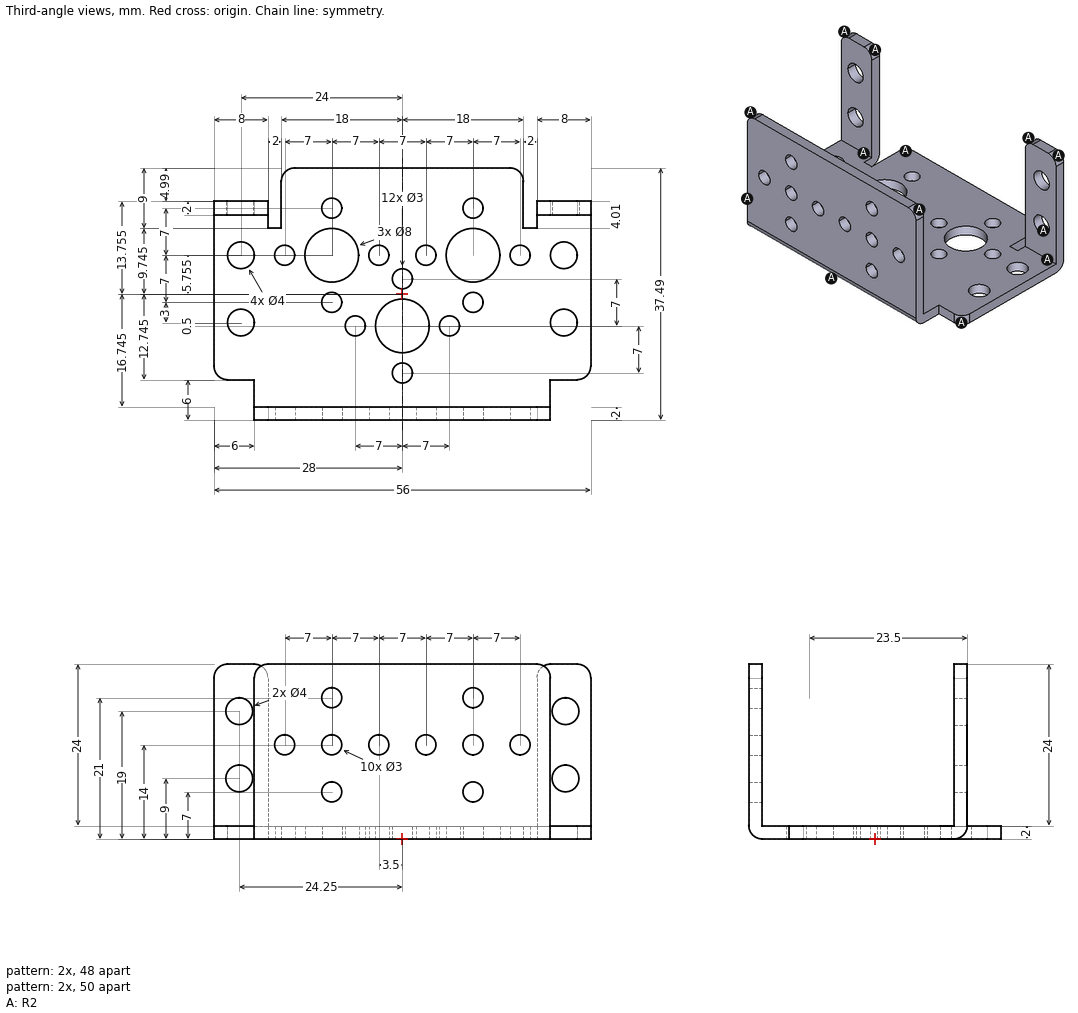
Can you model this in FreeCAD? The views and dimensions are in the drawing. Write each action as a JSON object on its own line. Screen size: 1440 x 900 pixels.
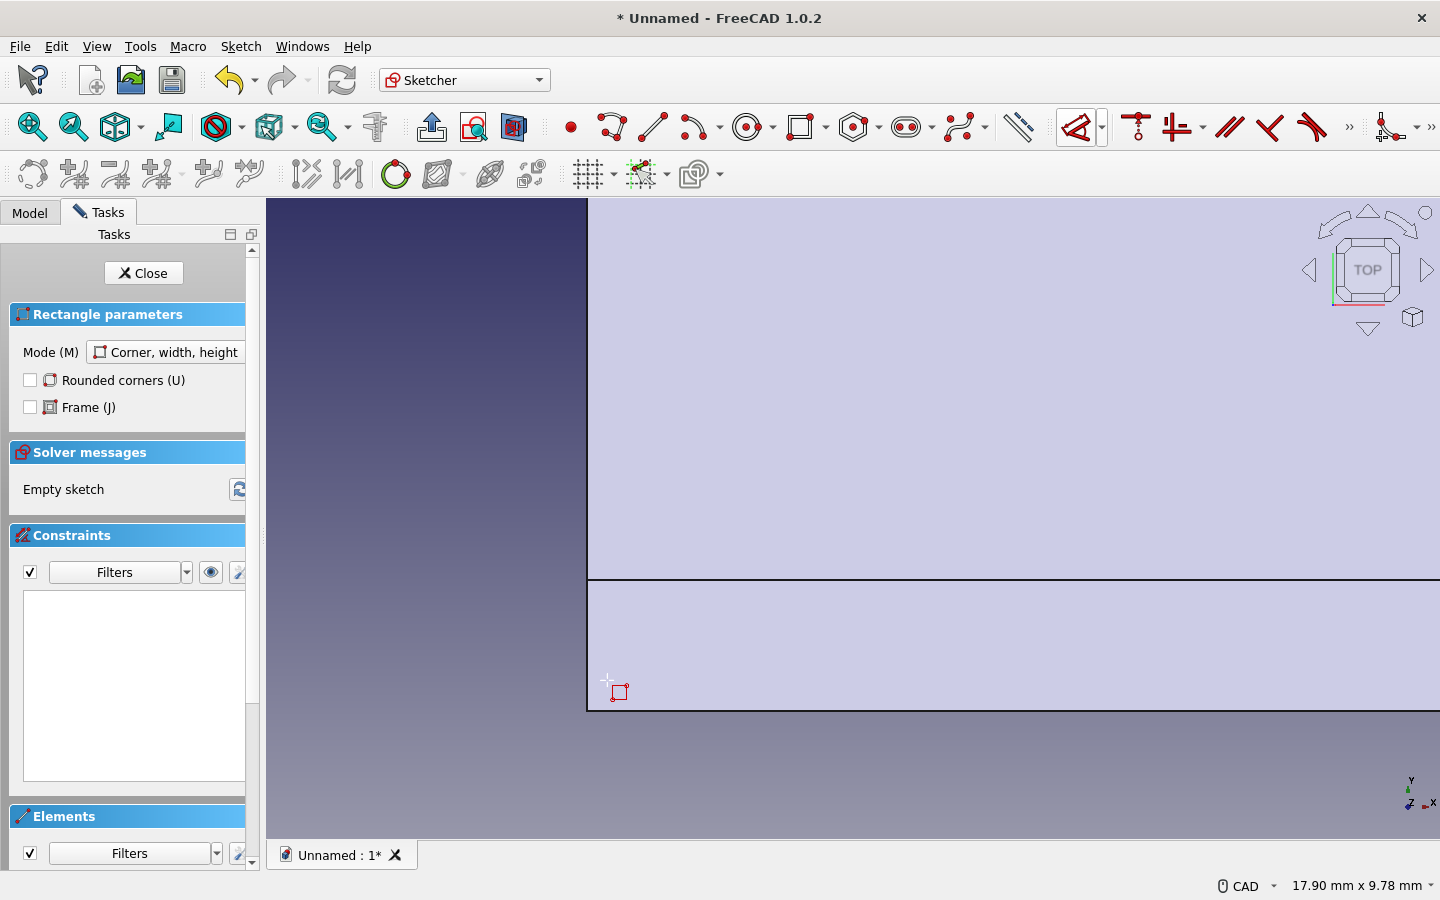
{"action": "left_click", "coordinate": [587, 318]}
{"action": "mouse_move", "coordinate": [980, 711]}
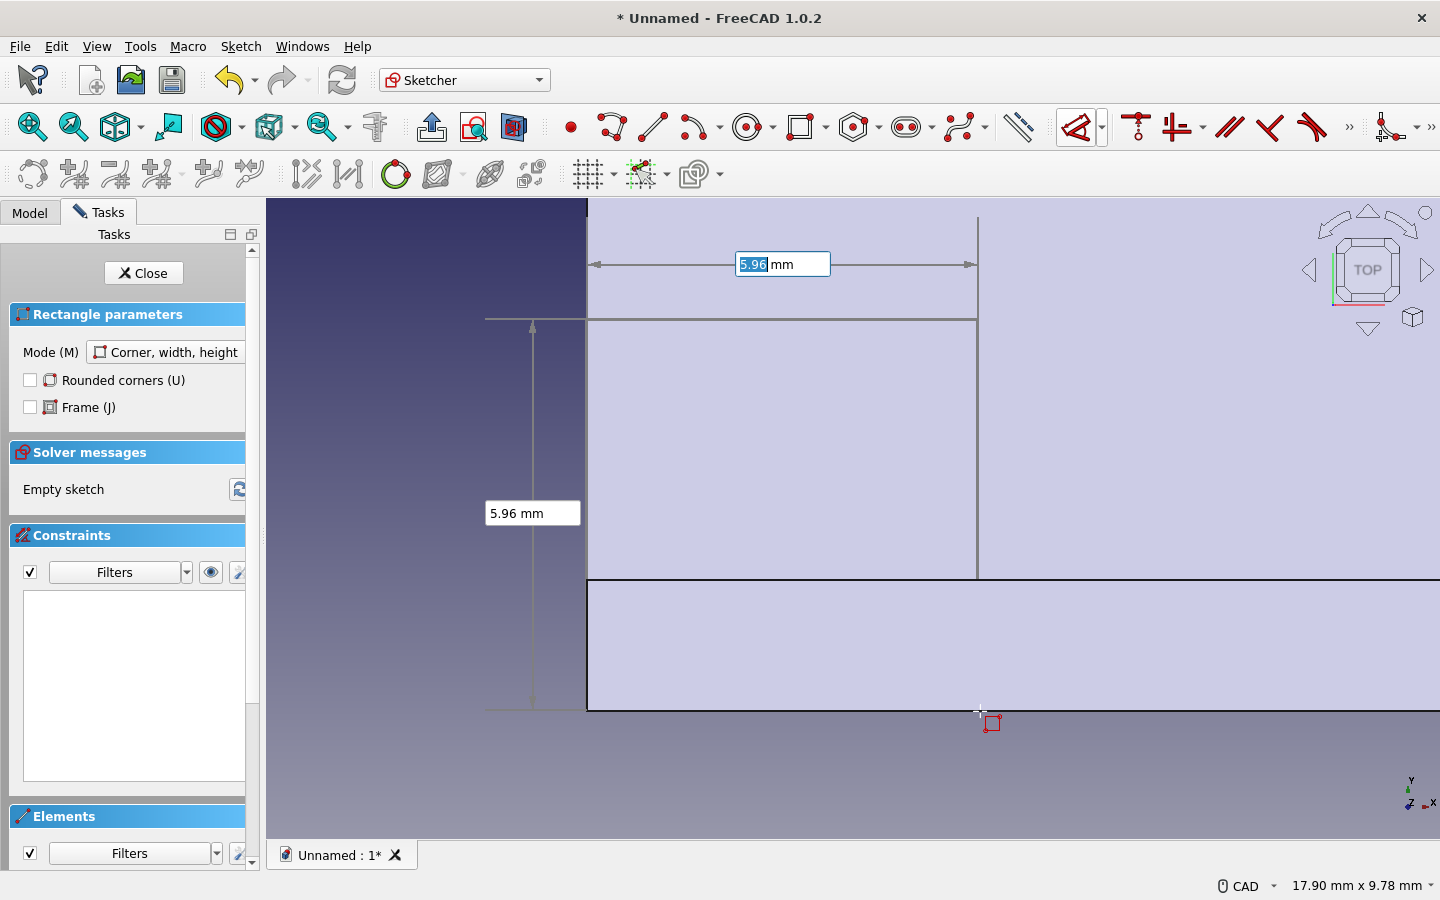
{"action": "type", "text": "6"}
{"action": "key", "text": "Tab"}
{"action": "type", "text": "6"}
{"action": "key", "text": "Return"}
{"action": "key", "text": "Escape"}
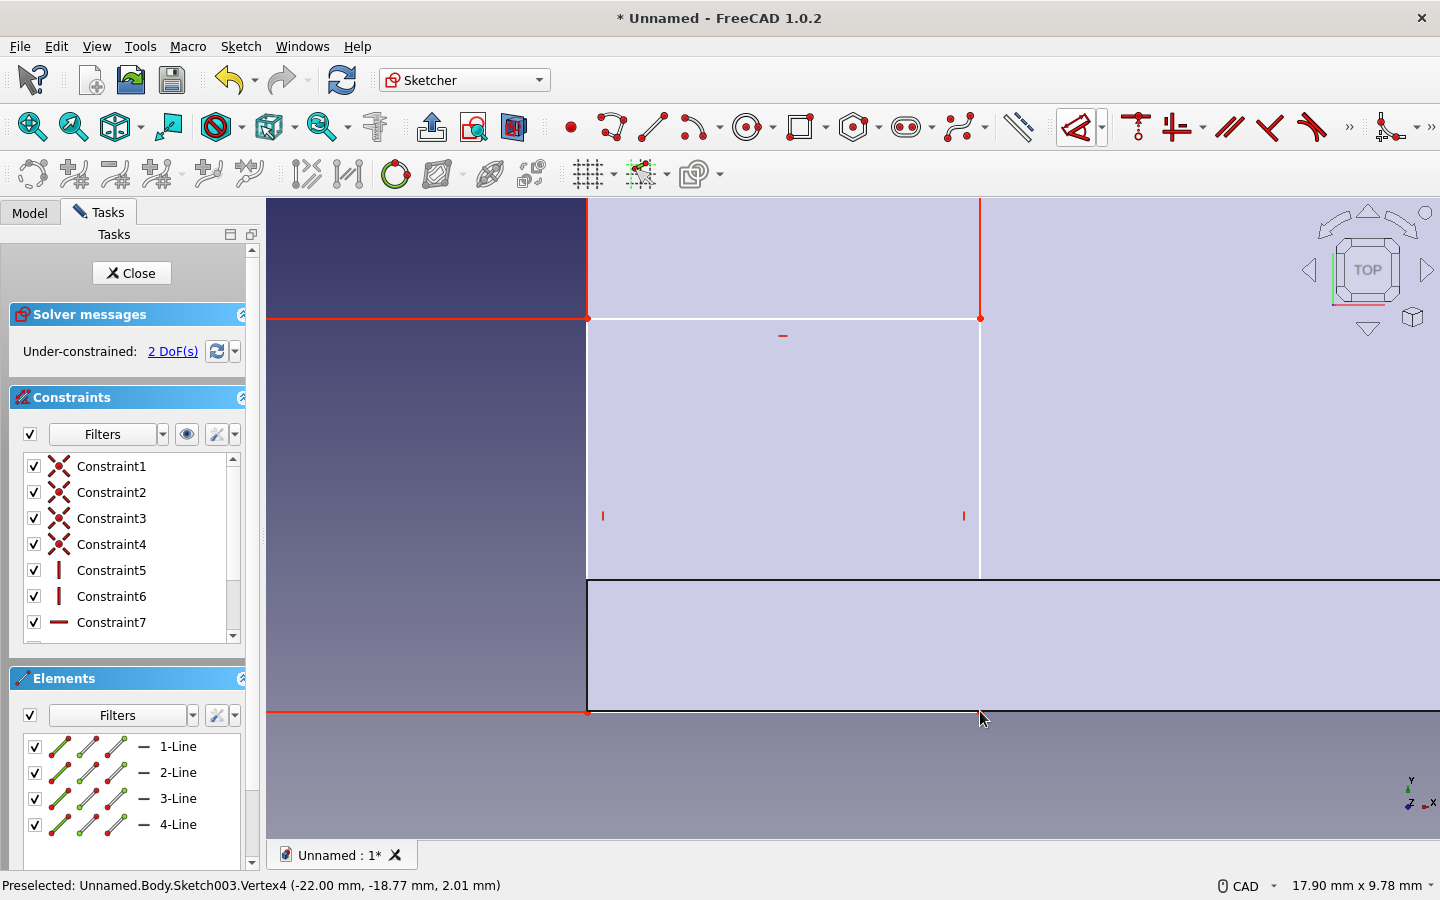
{"action": "left_click", "coordinate": [587, 319]}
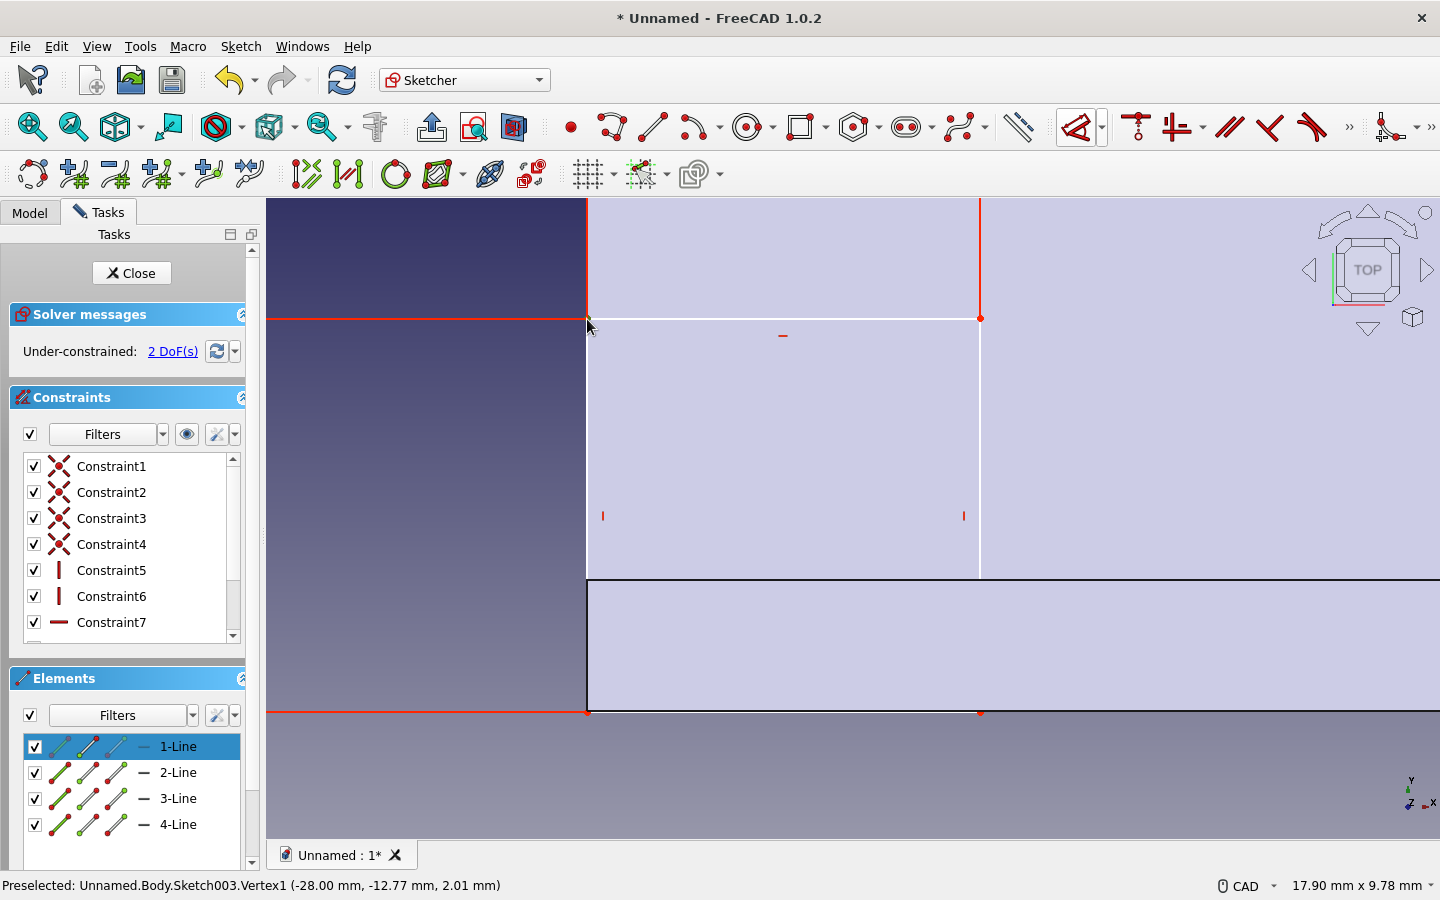
{"action": "key", "text": "l"}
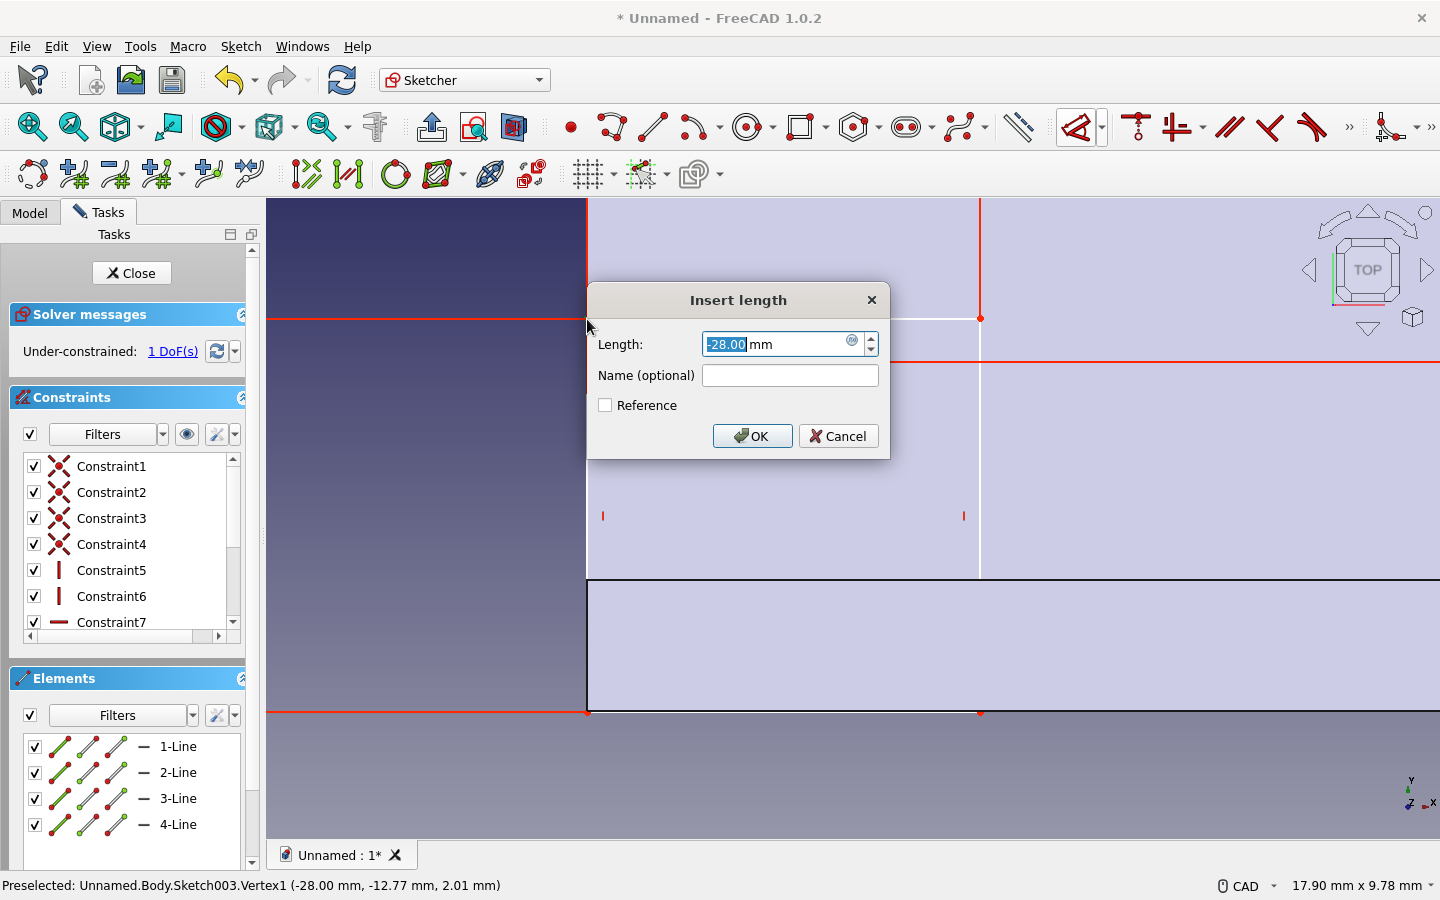
{"action": "type", "text": "-28"}
{"action": "key", "text": "Return"}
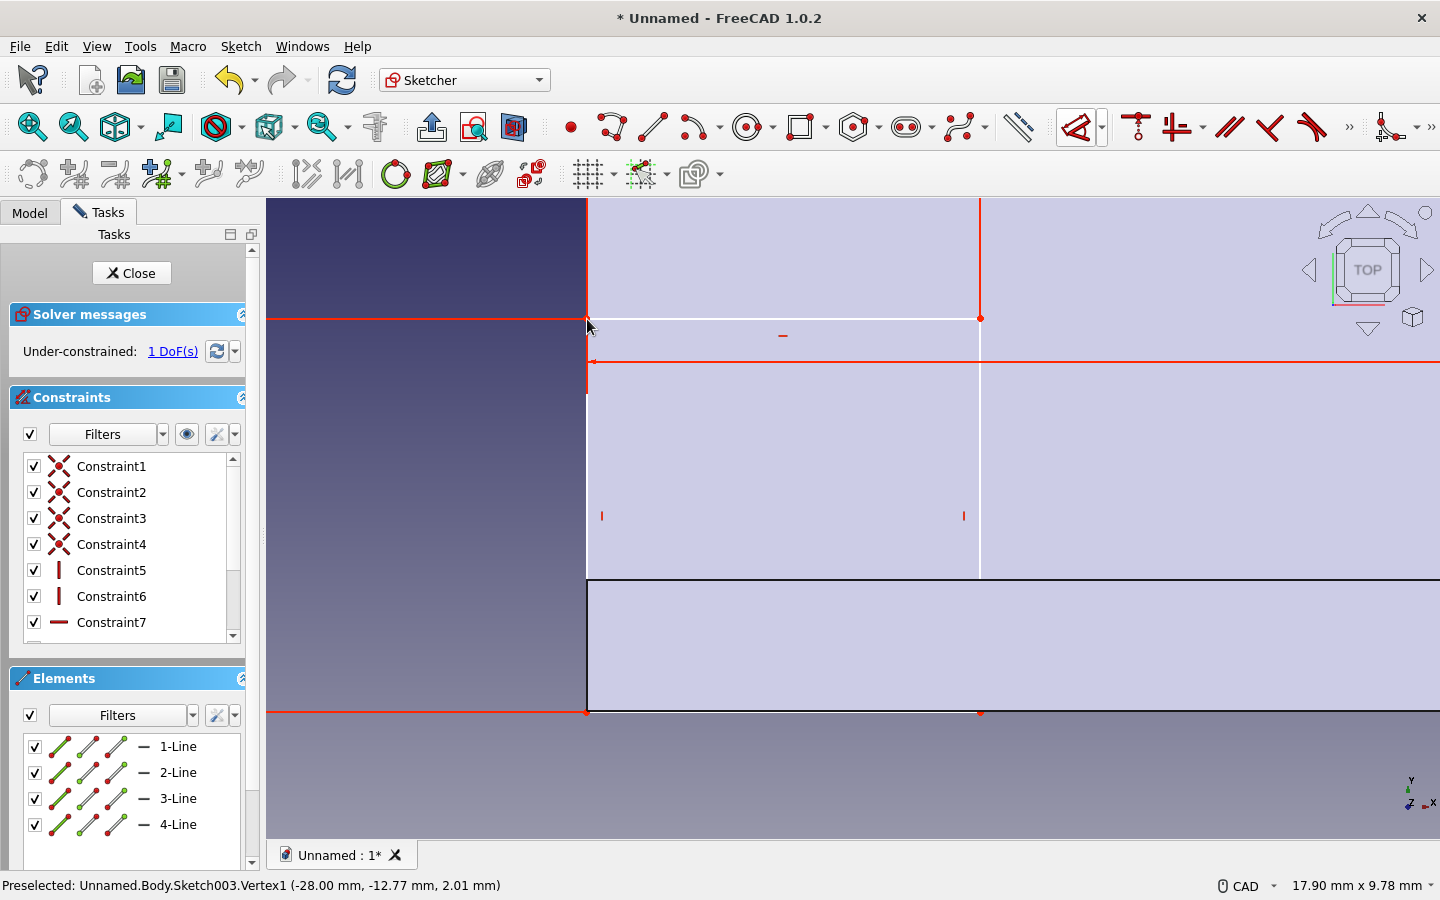
{"action": "left_click", "coordinate": [587, 319]}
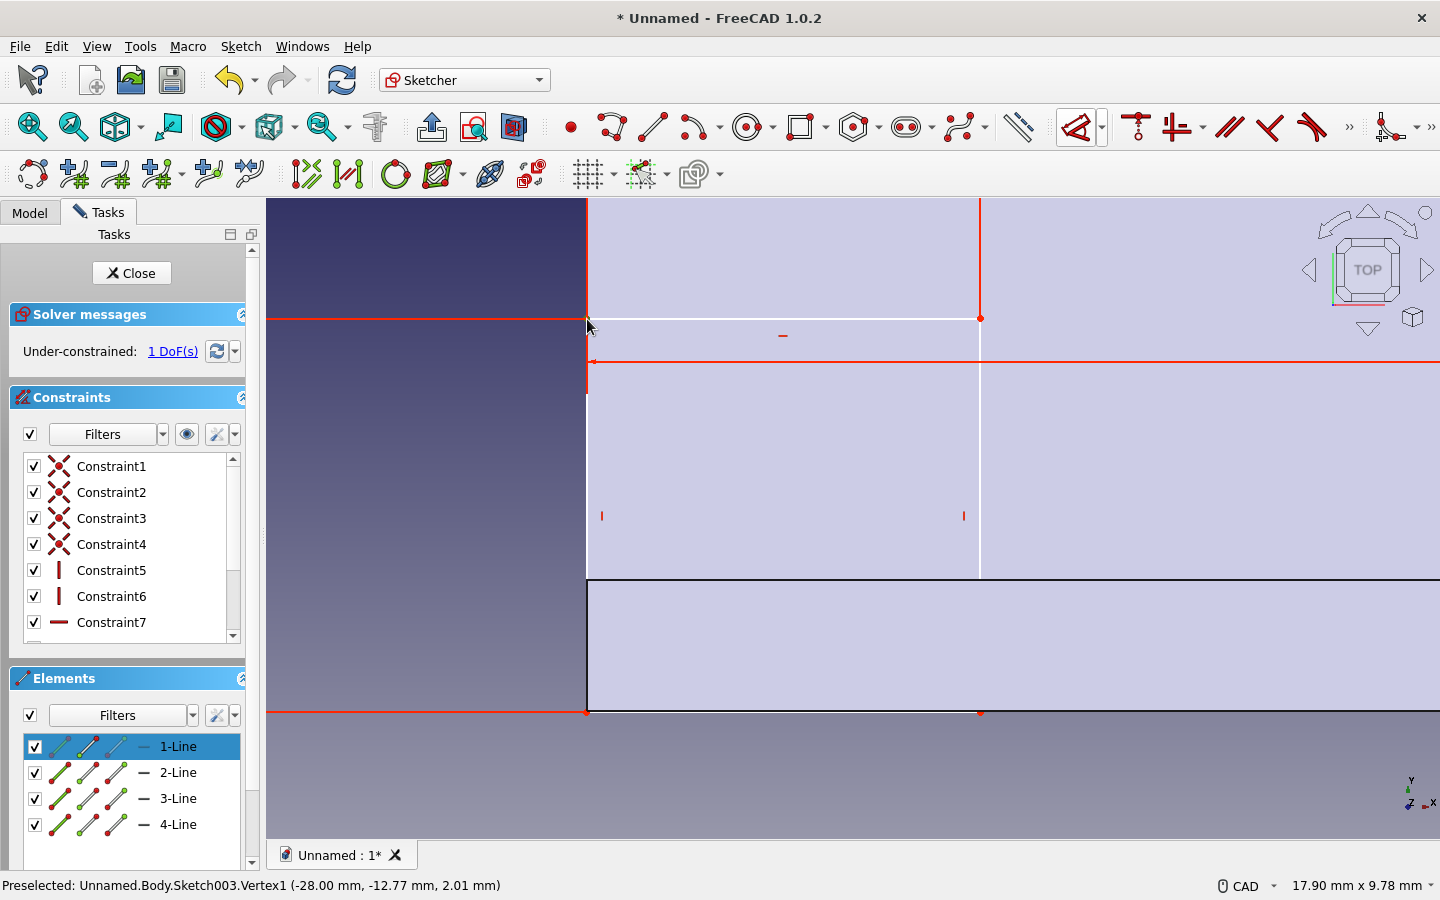
{"action": "key", "text": "i"}